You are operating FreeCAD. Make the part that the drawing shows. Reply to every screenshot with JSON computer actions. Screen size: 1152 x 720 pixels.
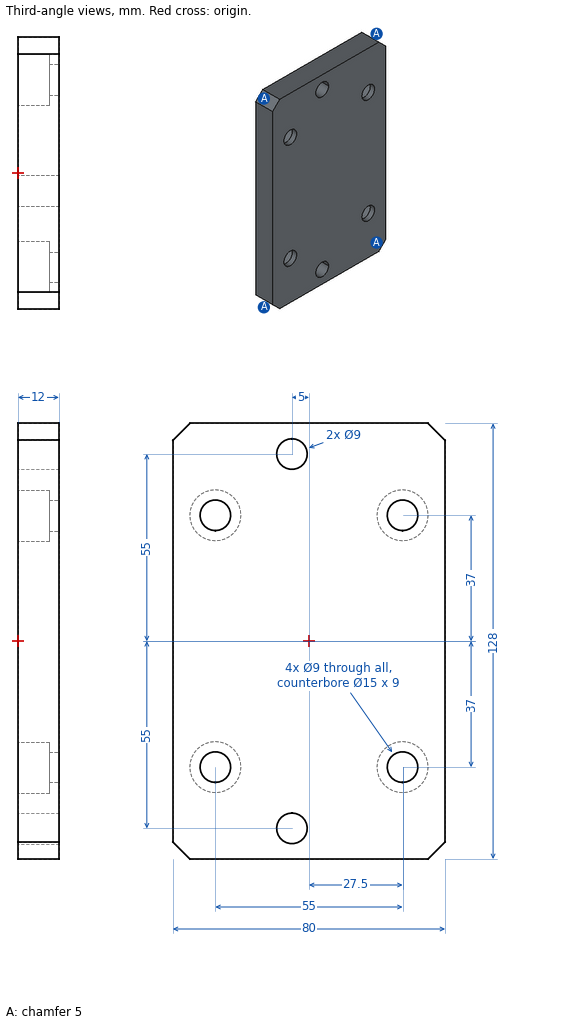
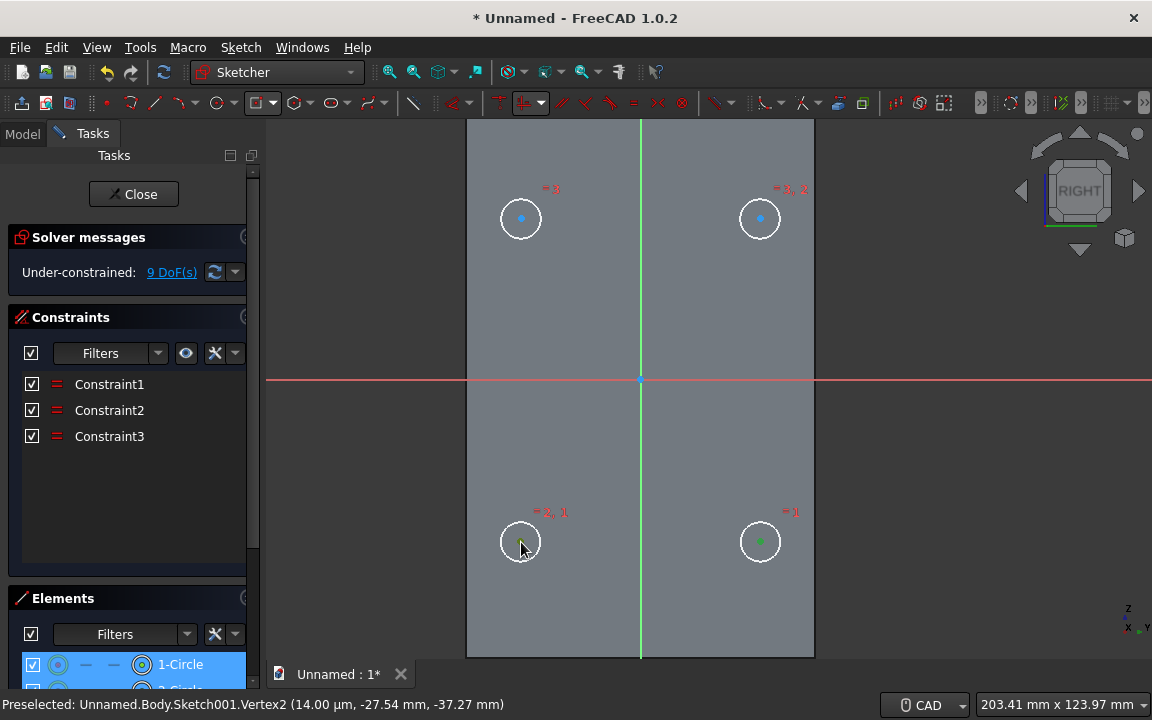
{"action": "key", "text": "h"}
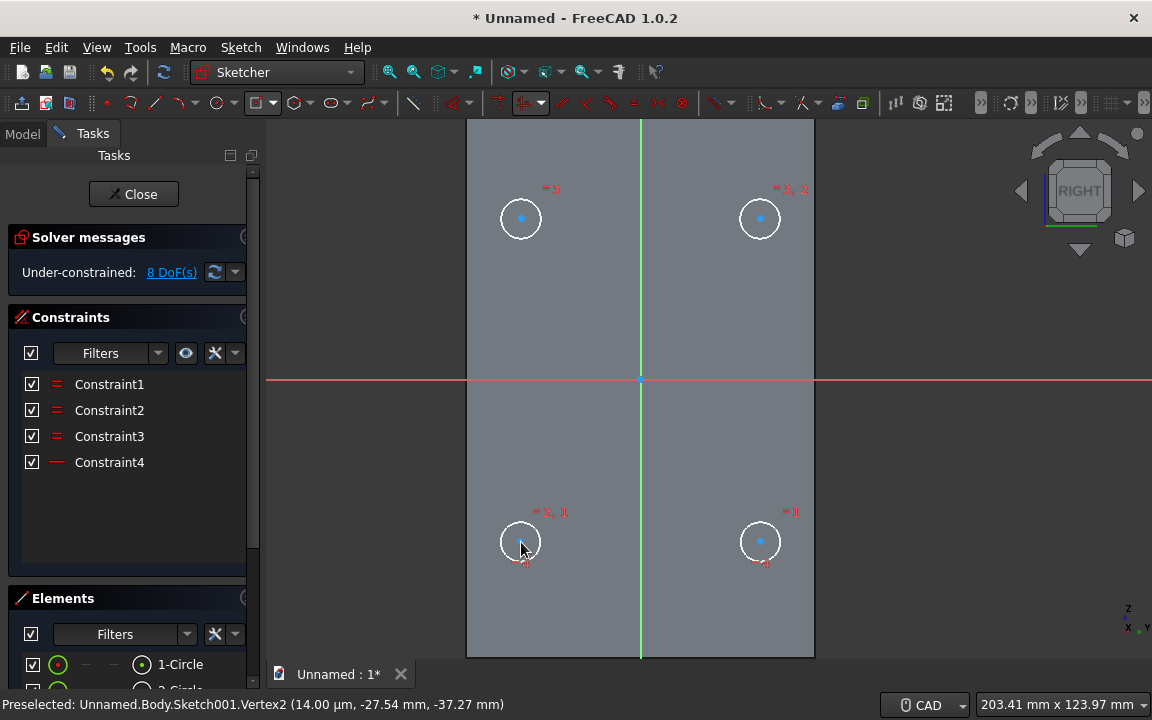
{"action": "left_click", "coordinate": [760, 542]}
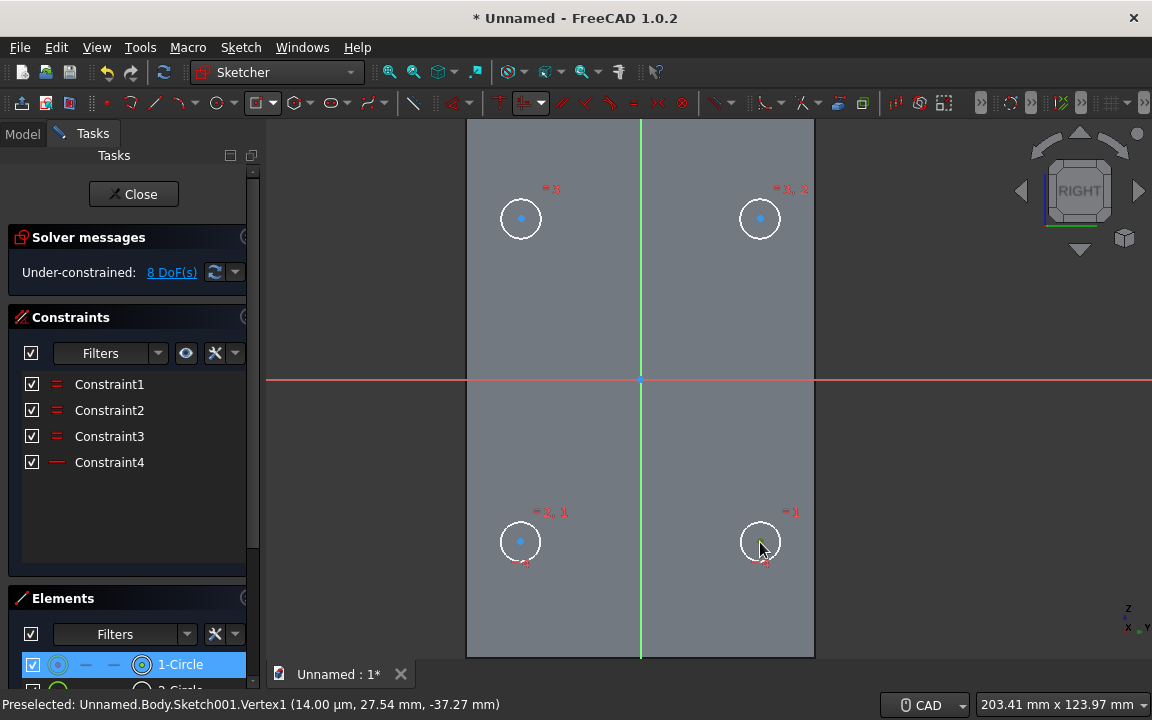
{"action": "left_click", "coordinate": [760, 219]}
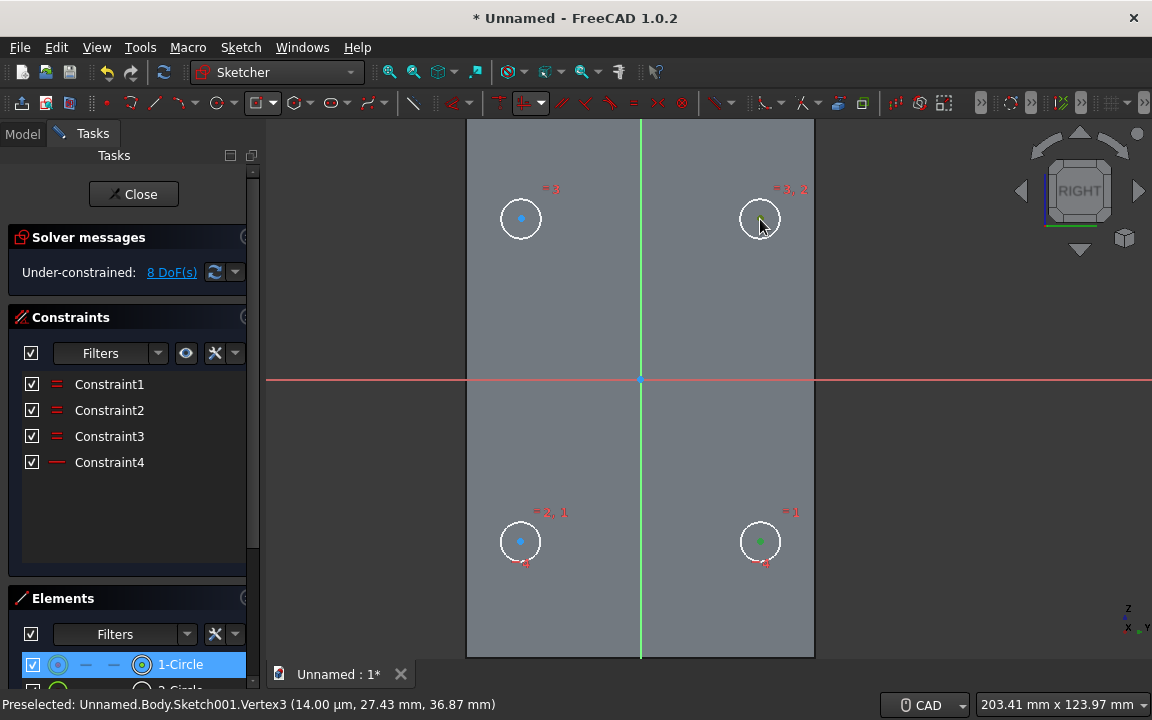
{"action": "left_click", "coordinate": [544, 104]}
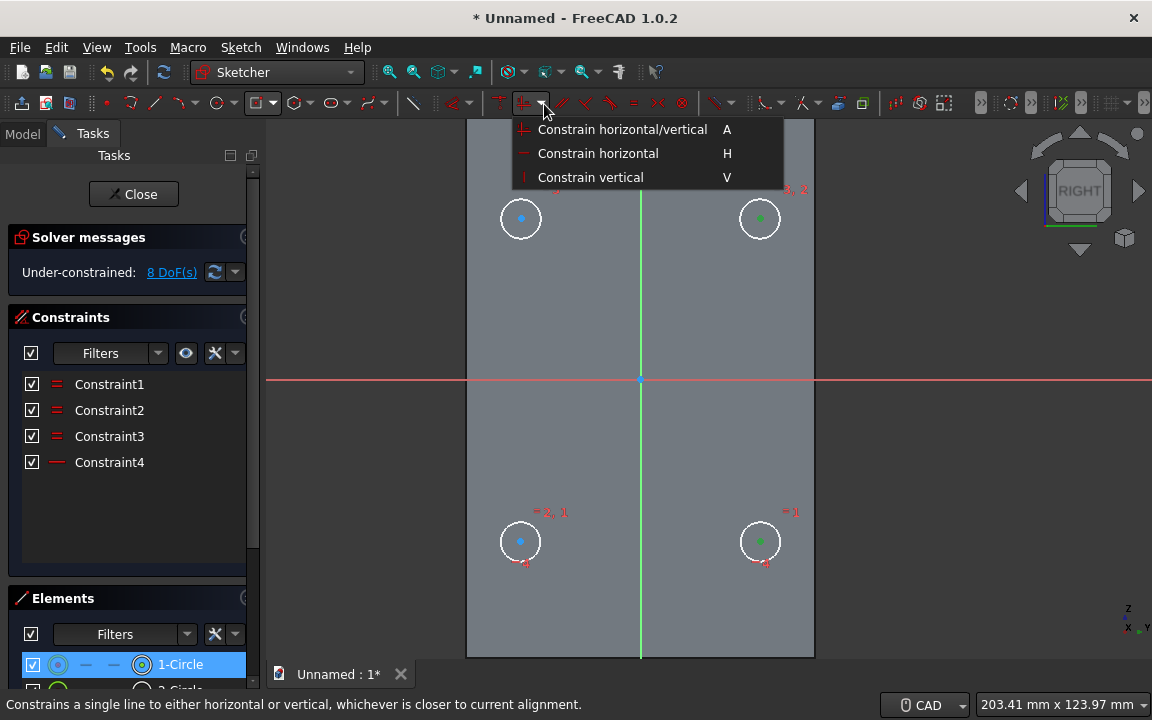
{"action": "left_click", "coordinate": [648, 177]}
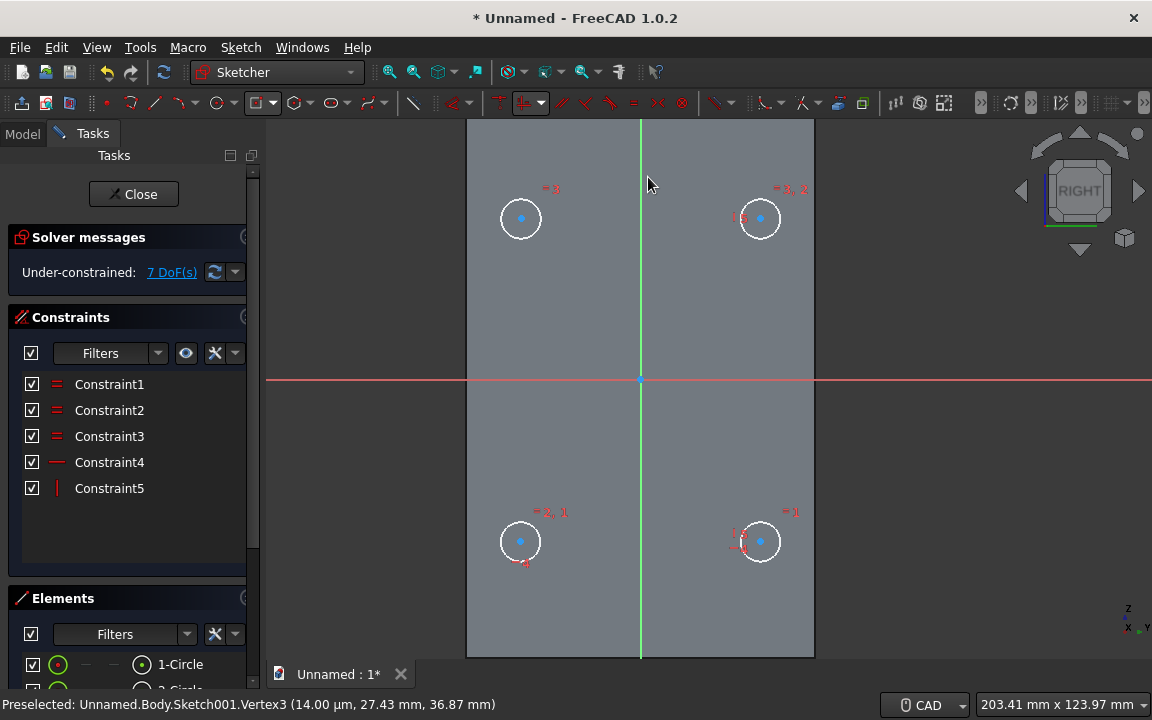
{"action": "left_click", "coordinate": [521, 542]}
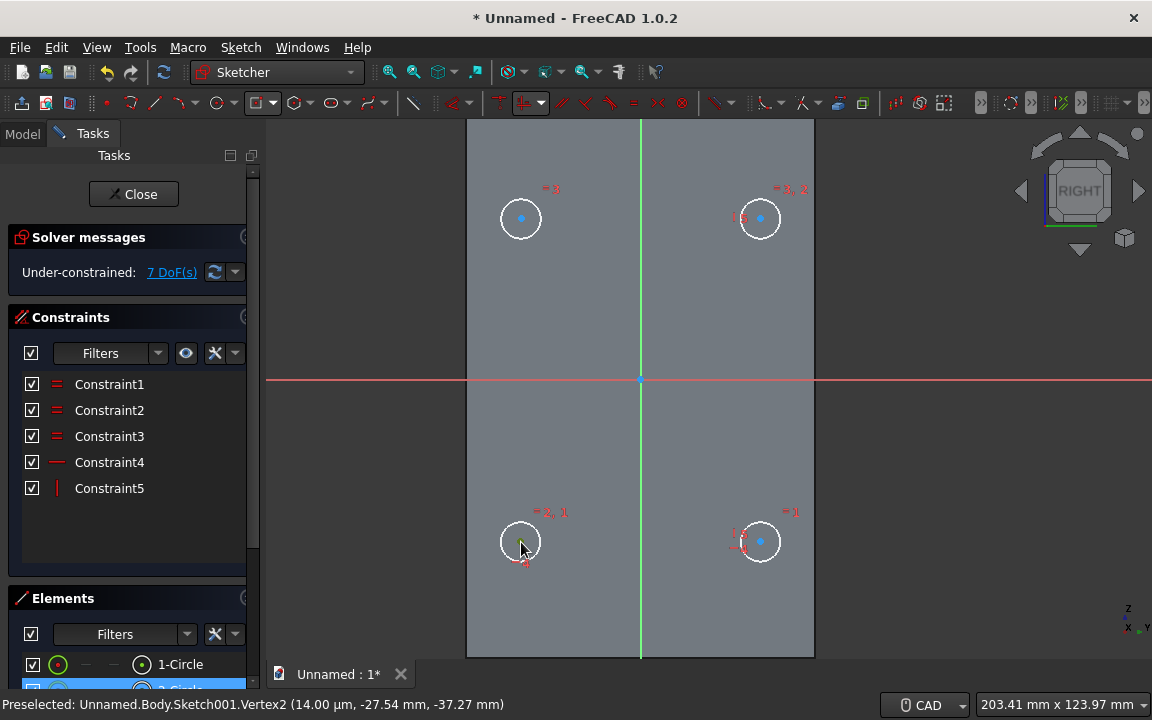
{"action": "left_click", "coordinate": [521, 219]}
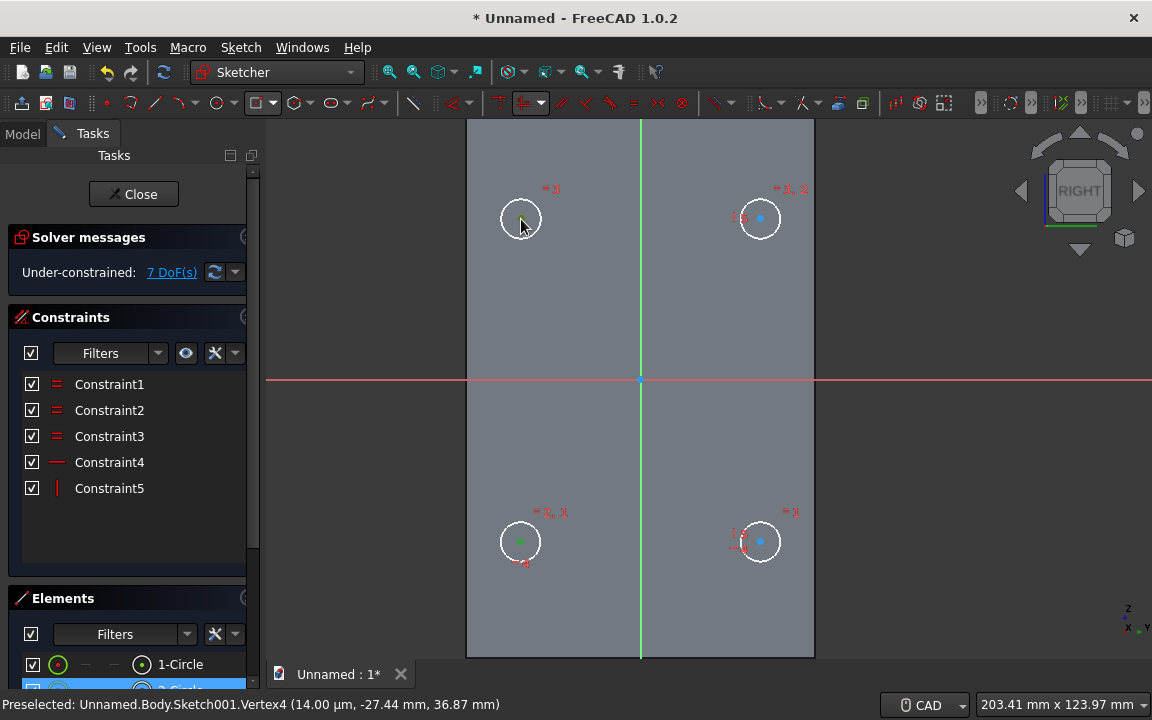
{"action": "key", "text": "v"}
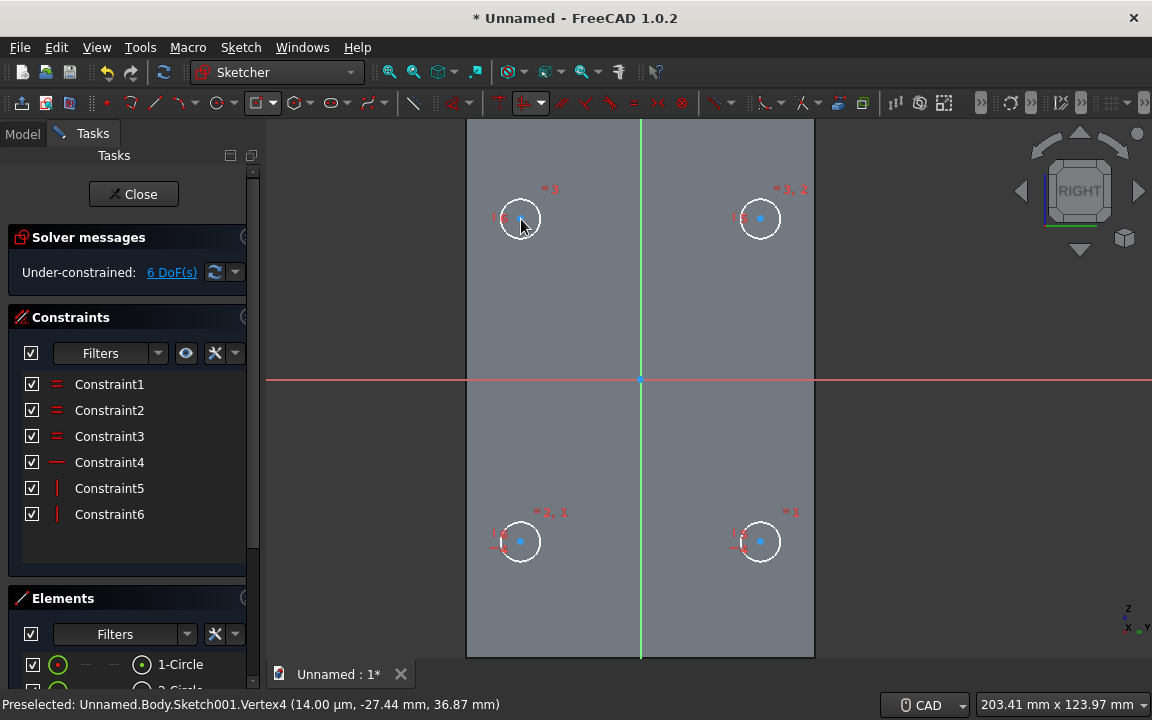
{"action": "left_click", "coordinate": [760, 219]}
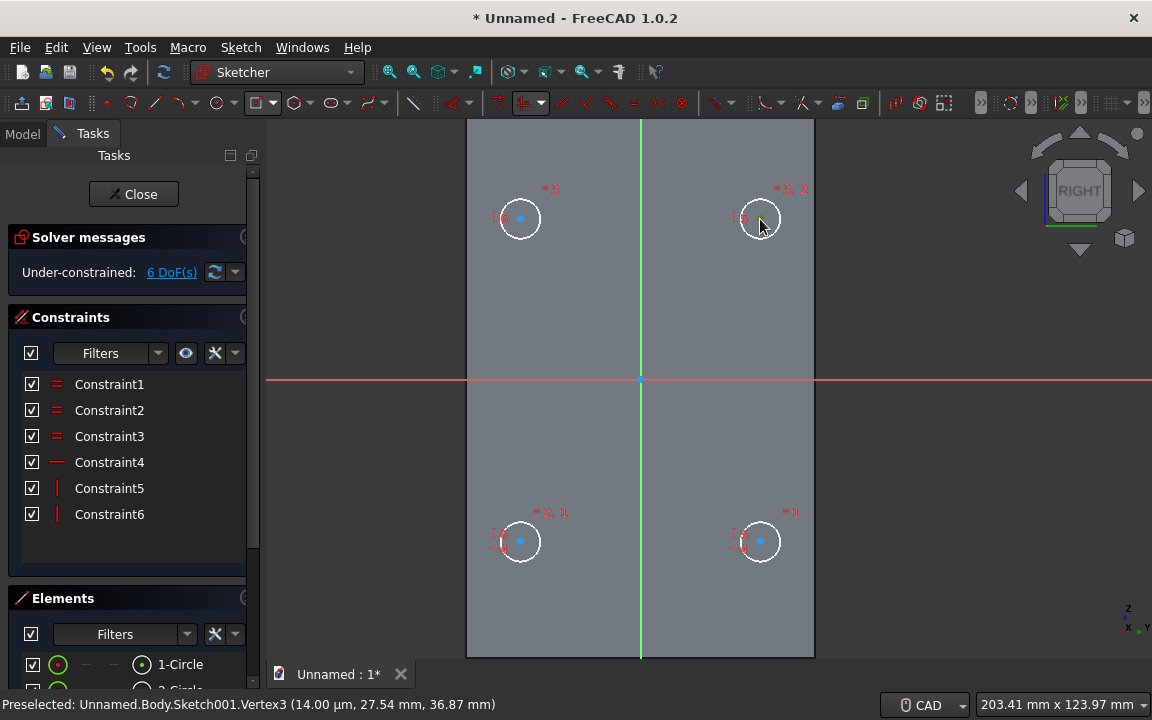
{"action": "left_click", "coordinate": [521, 219]}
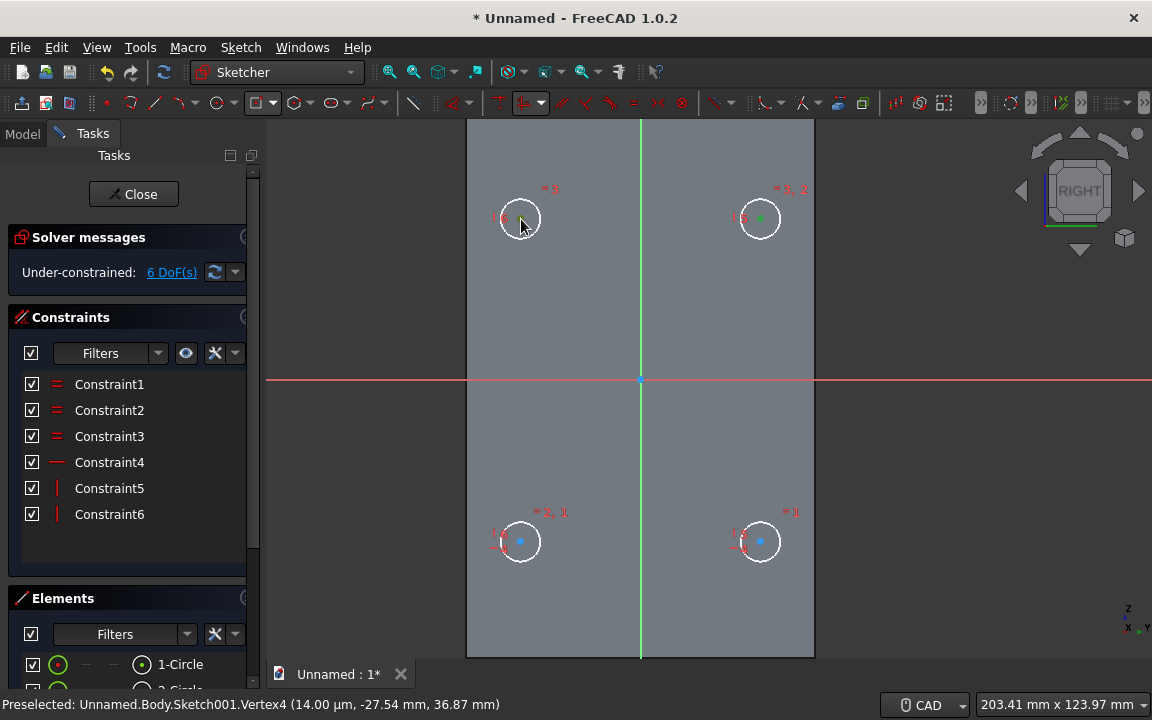
{"action": "left_click", "coordinate": [544, 104]}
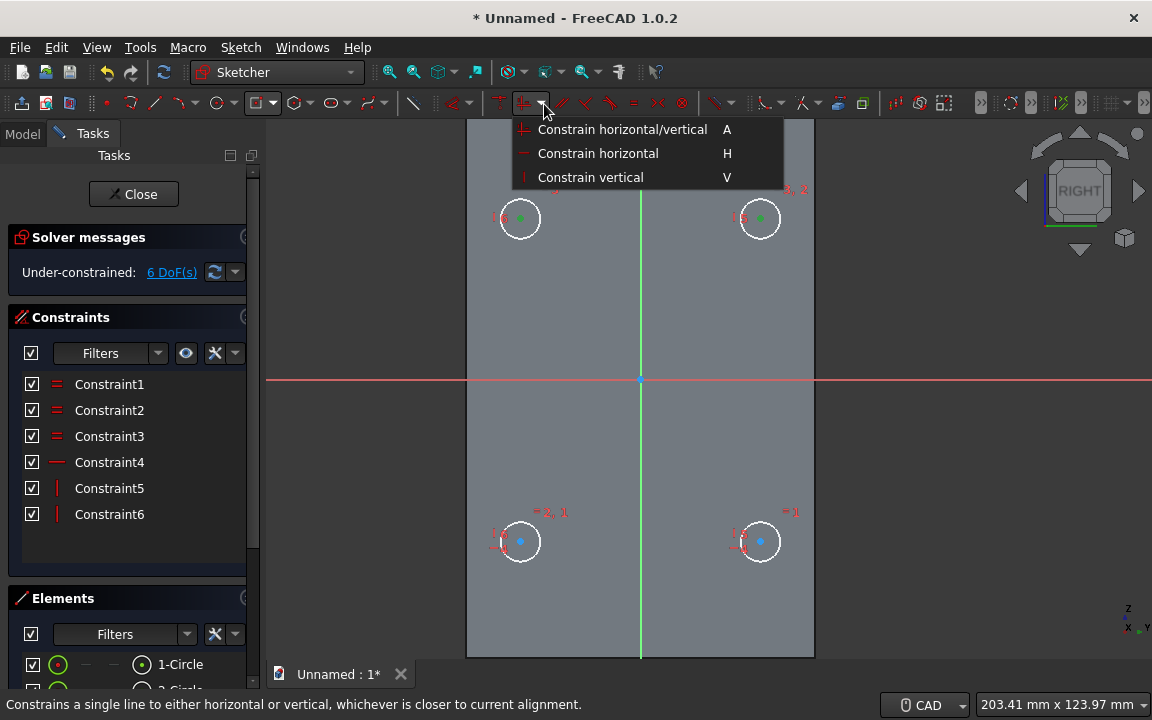
{"action": "left_click", "coordinate": [648, 153]}